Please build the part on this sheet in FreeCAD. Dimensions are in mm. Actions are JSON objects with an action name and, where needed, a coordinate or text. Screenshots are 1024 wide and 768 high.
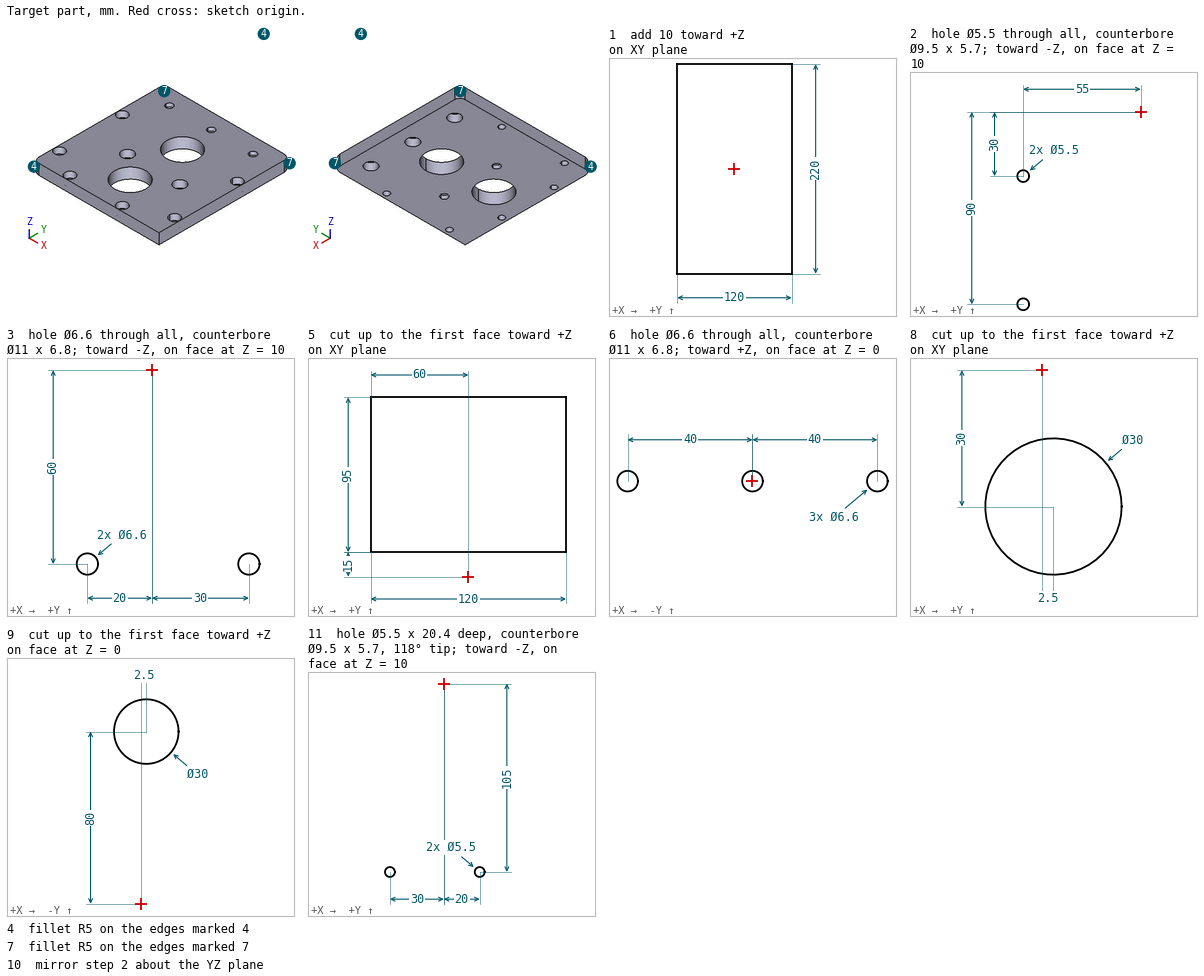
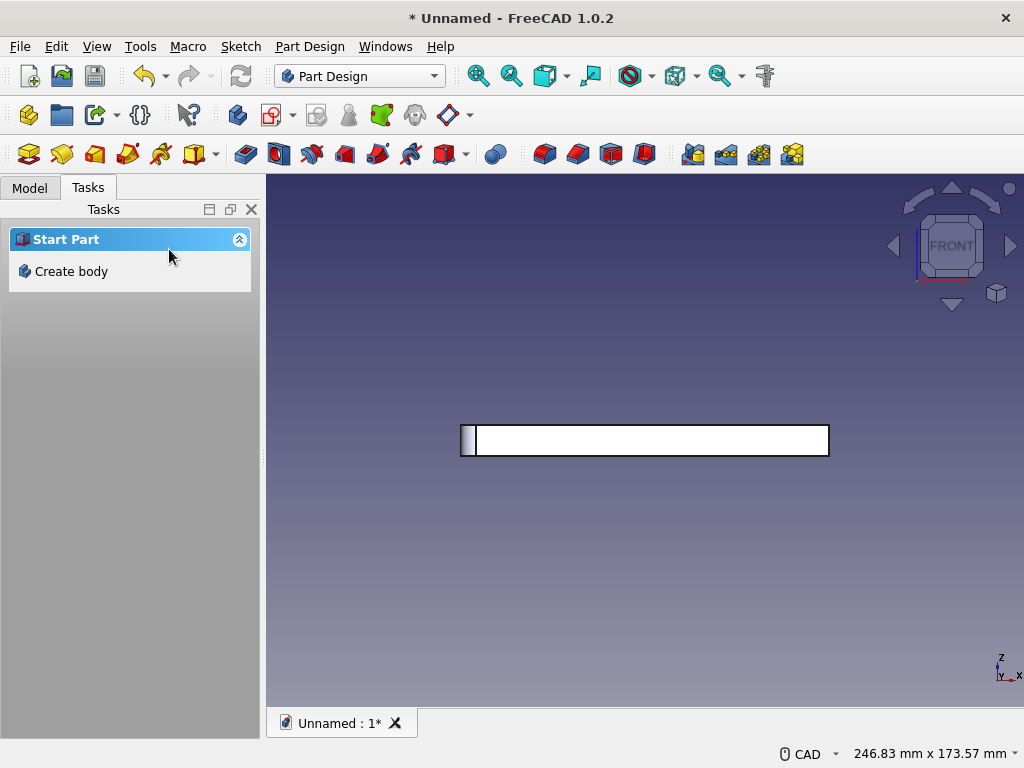
{"action": "key", "text": "3"}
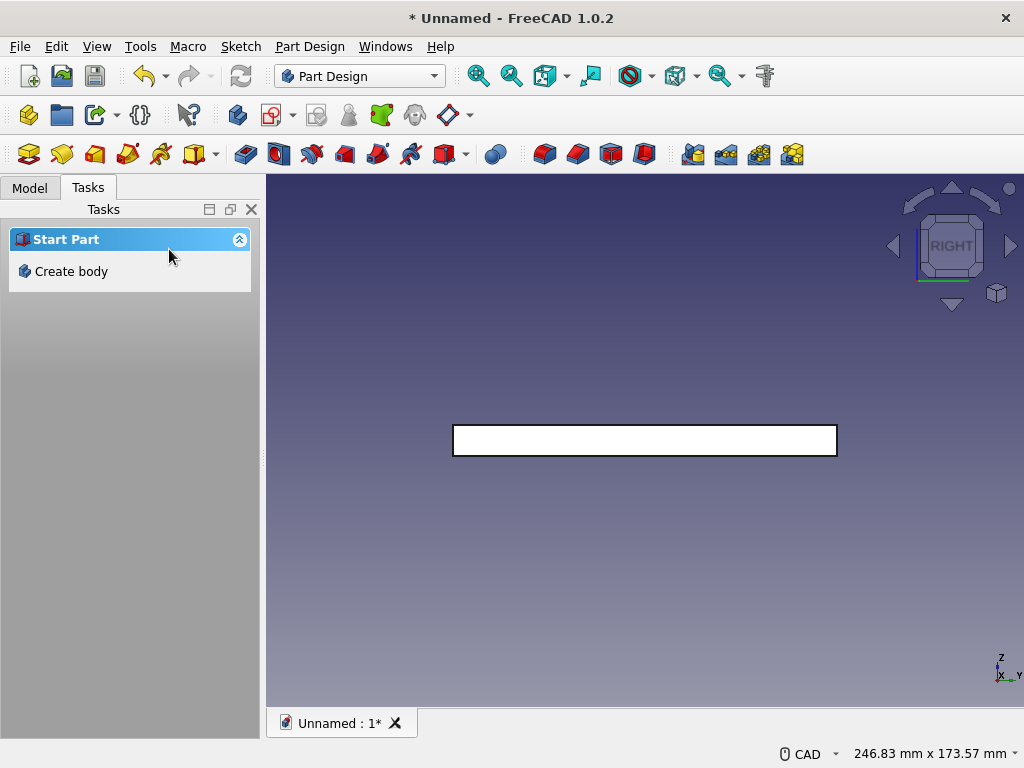
{"action": "left_click", "coordinate": [837, 439]}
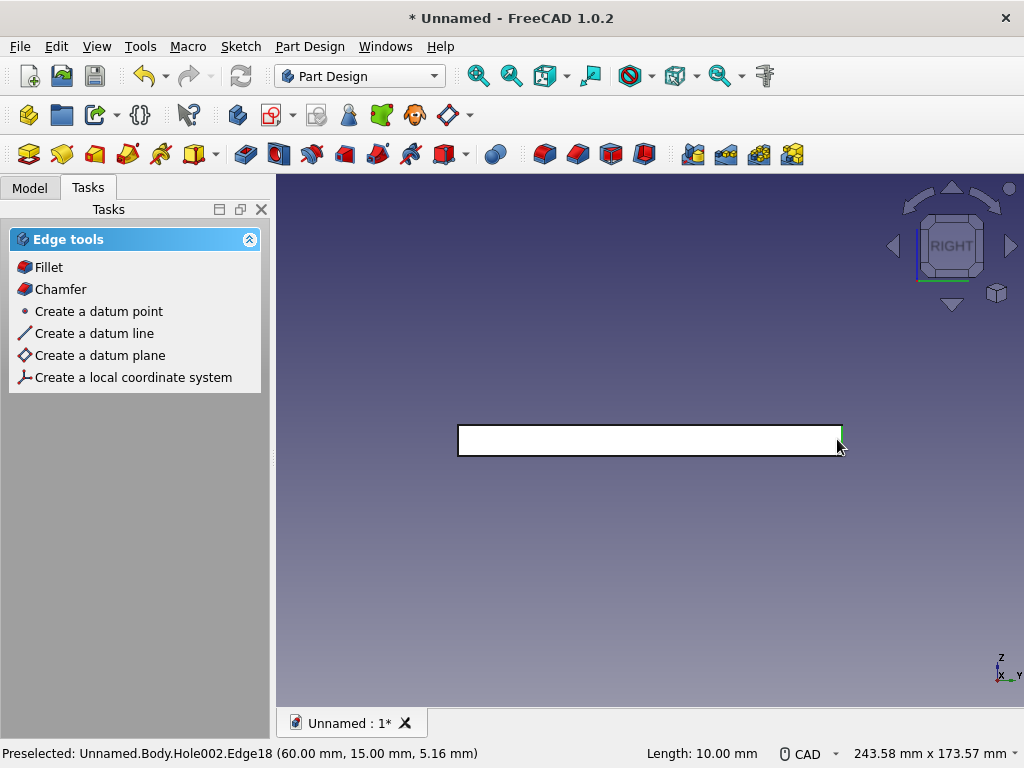
{"action": "key", "text": "5"}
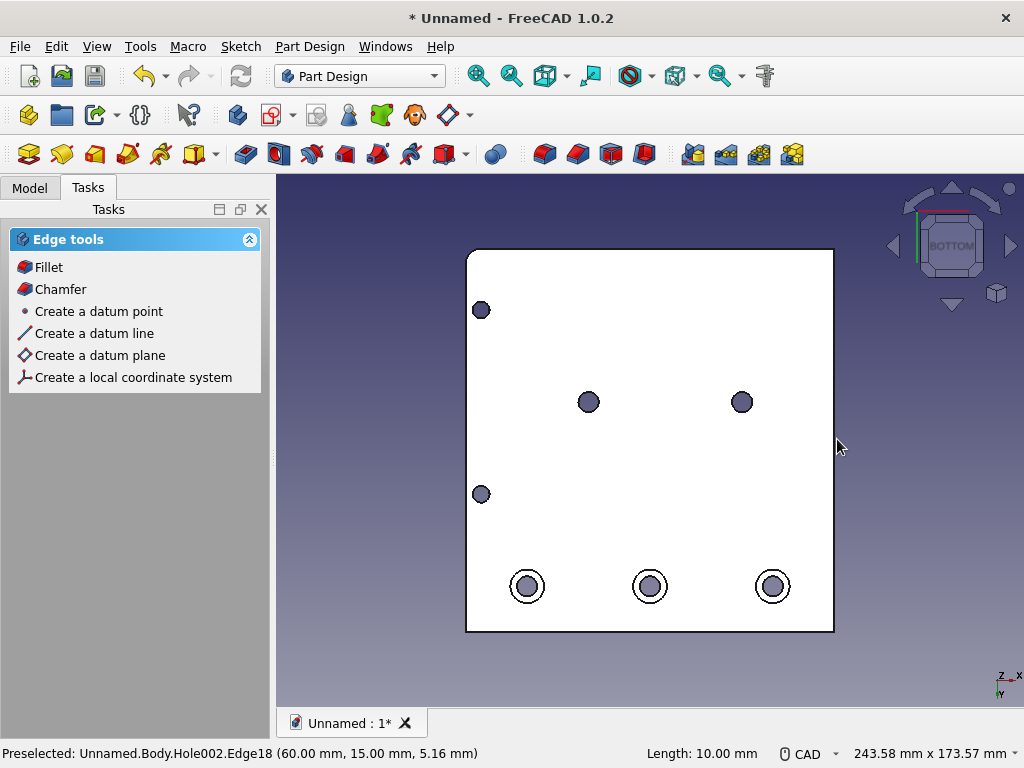
{"action": "key", "text": "4"}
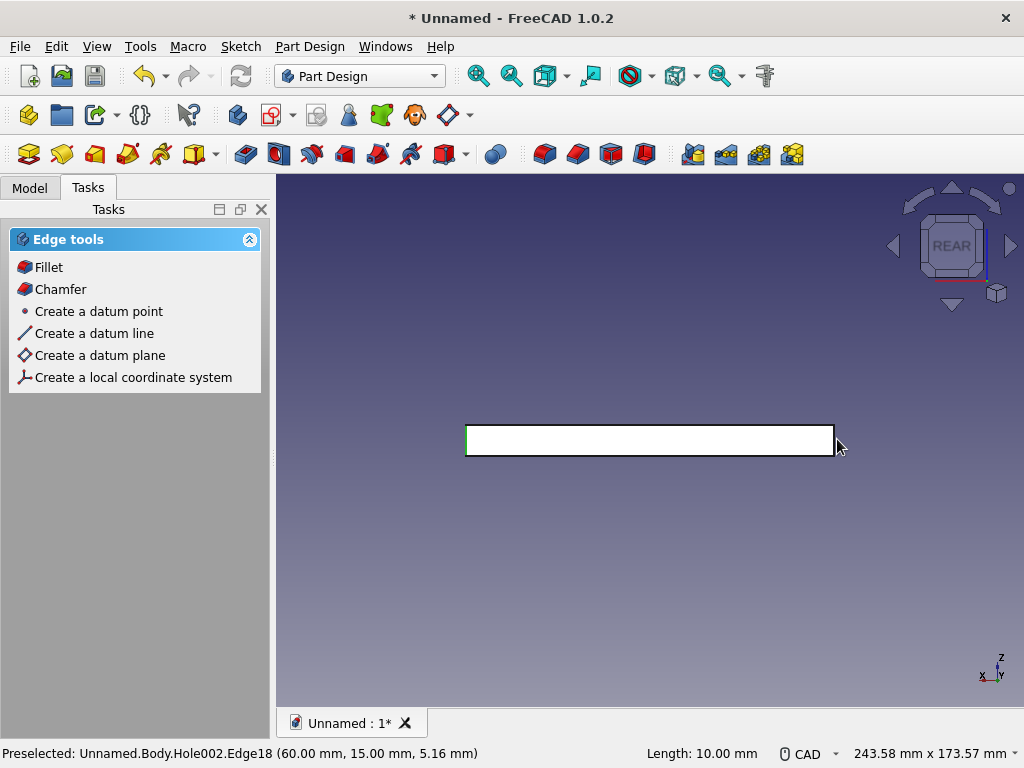
{"action": "left_click", "coordinate": [834, 439], "text": "ctrl"}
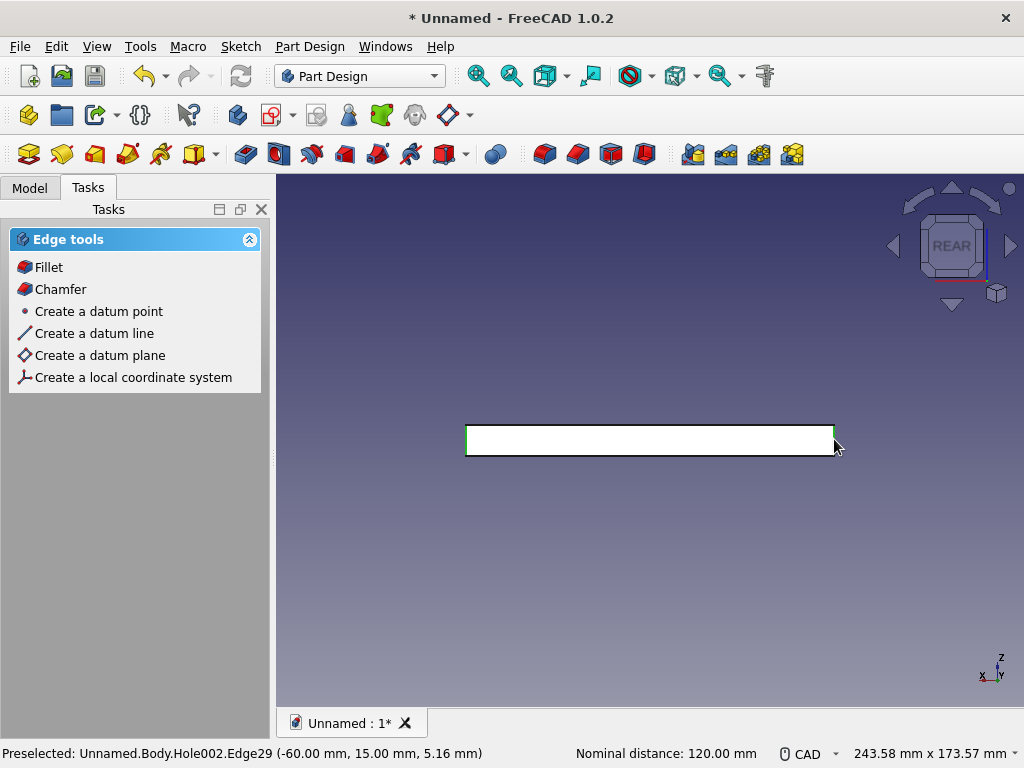
{"action": "left_click", "coordinate": [545, 154]}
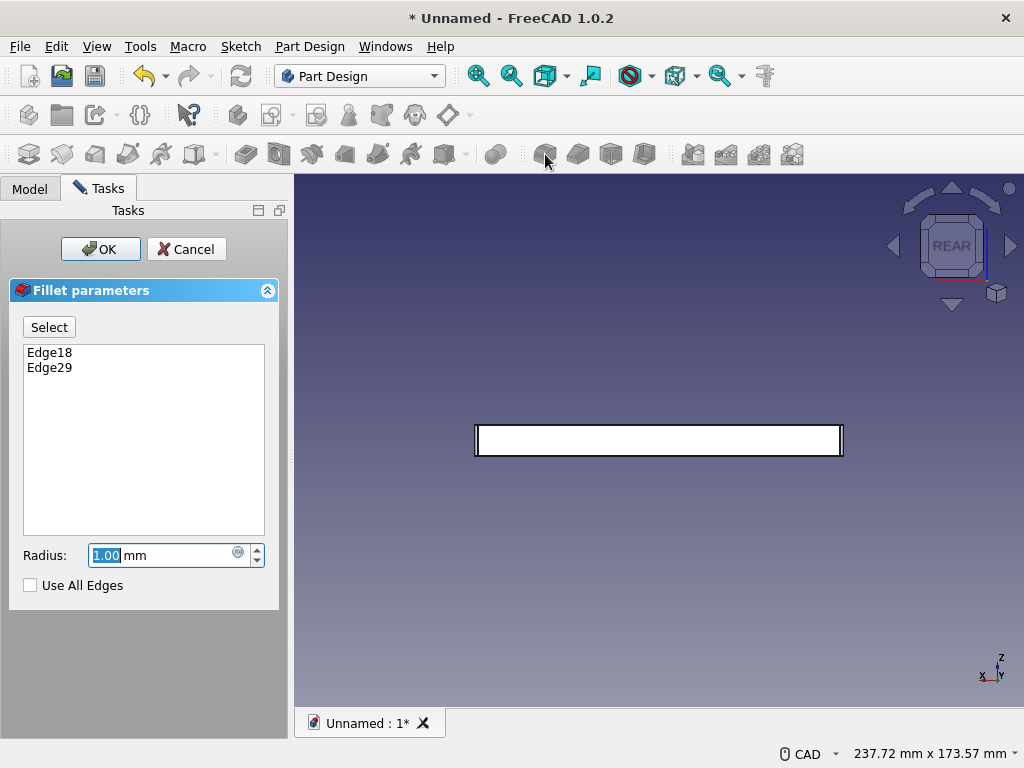
{"action": "type", "text": "5"}
{"action": "key", "text": "Tab"}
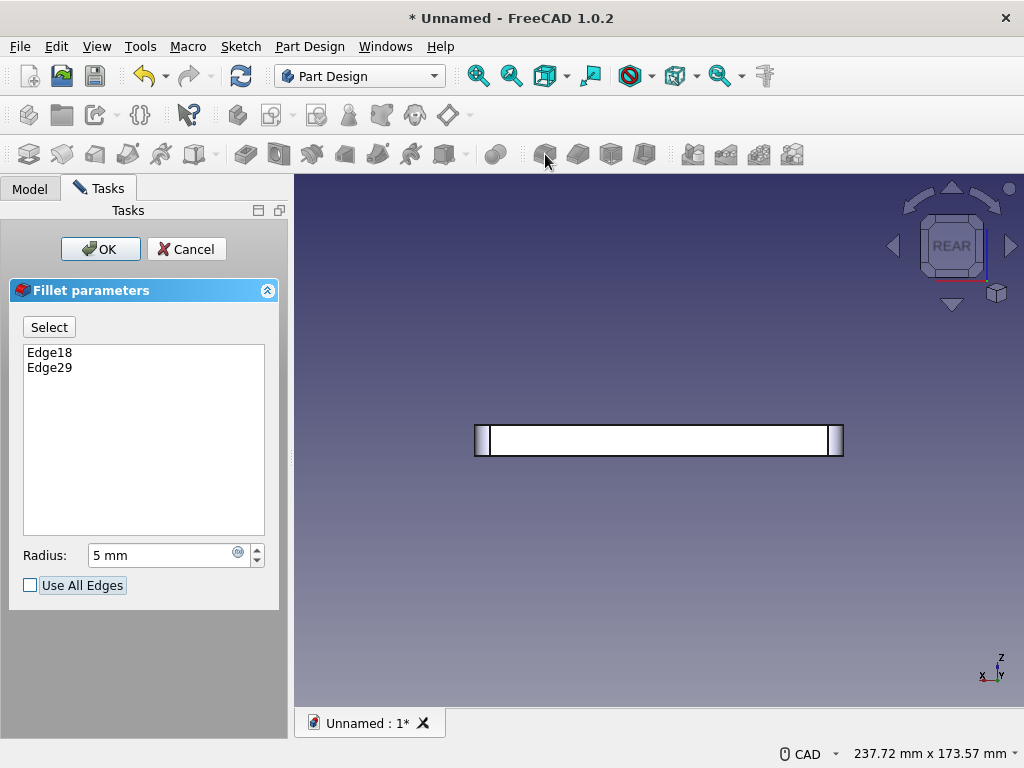
{"action": "left_click", "coordinate": [101, 249]}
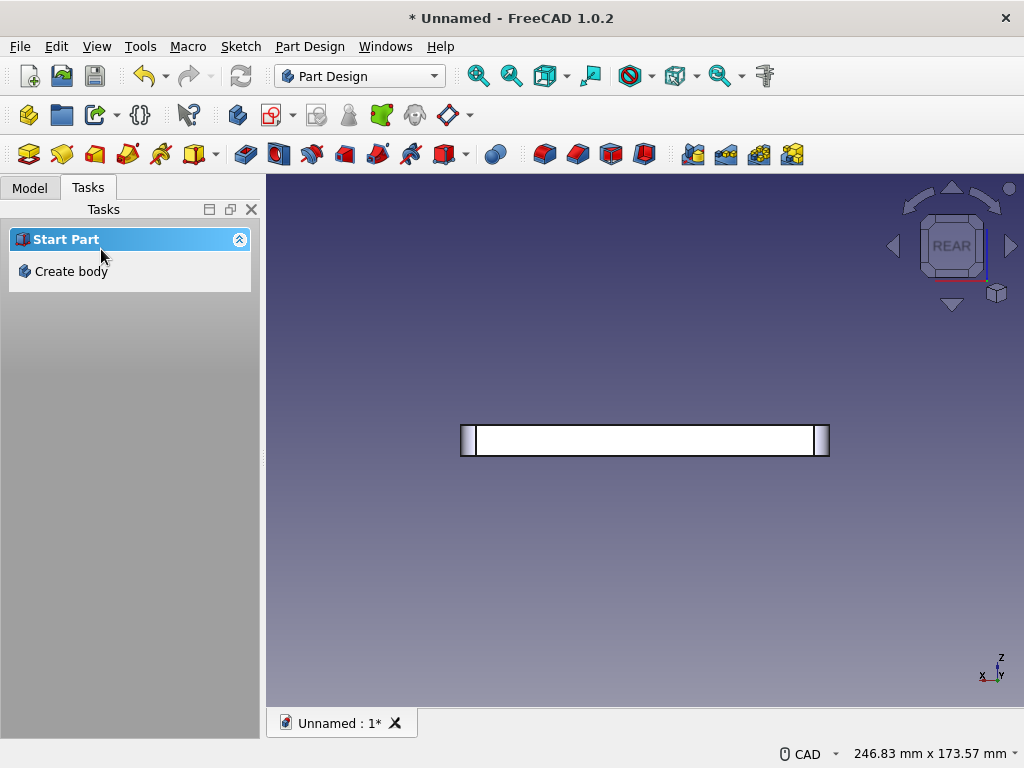
{"action": "left_click", "coordinate": [270, 116]}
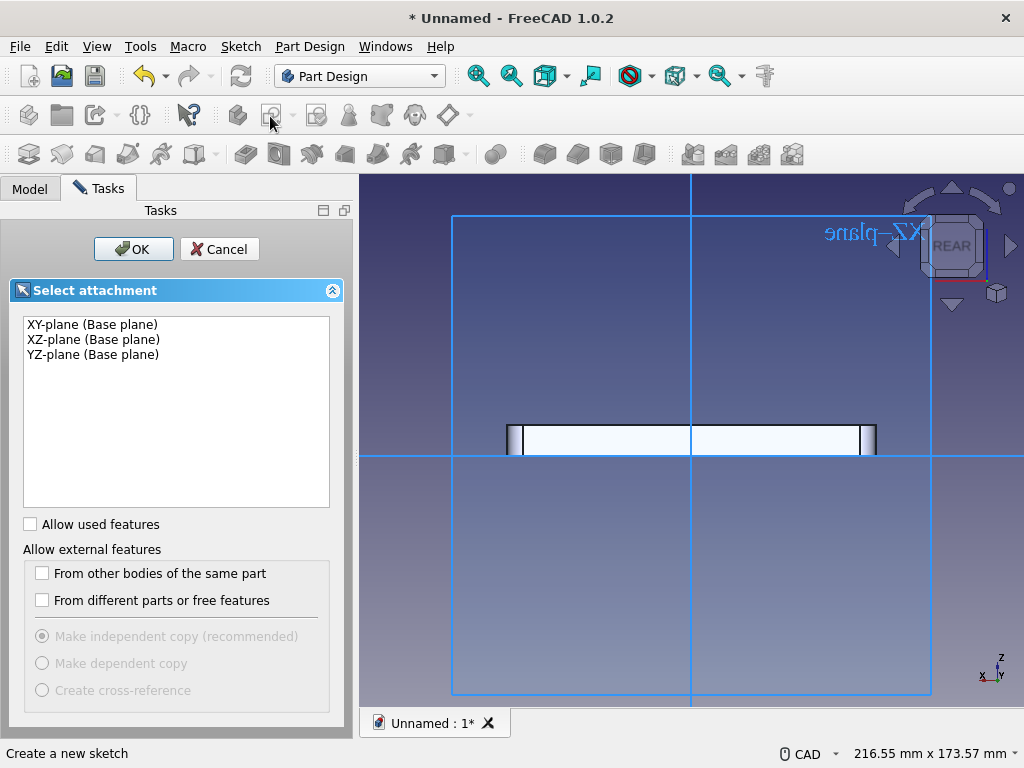
{"action": "left_click", "coordinate": [84, 324]}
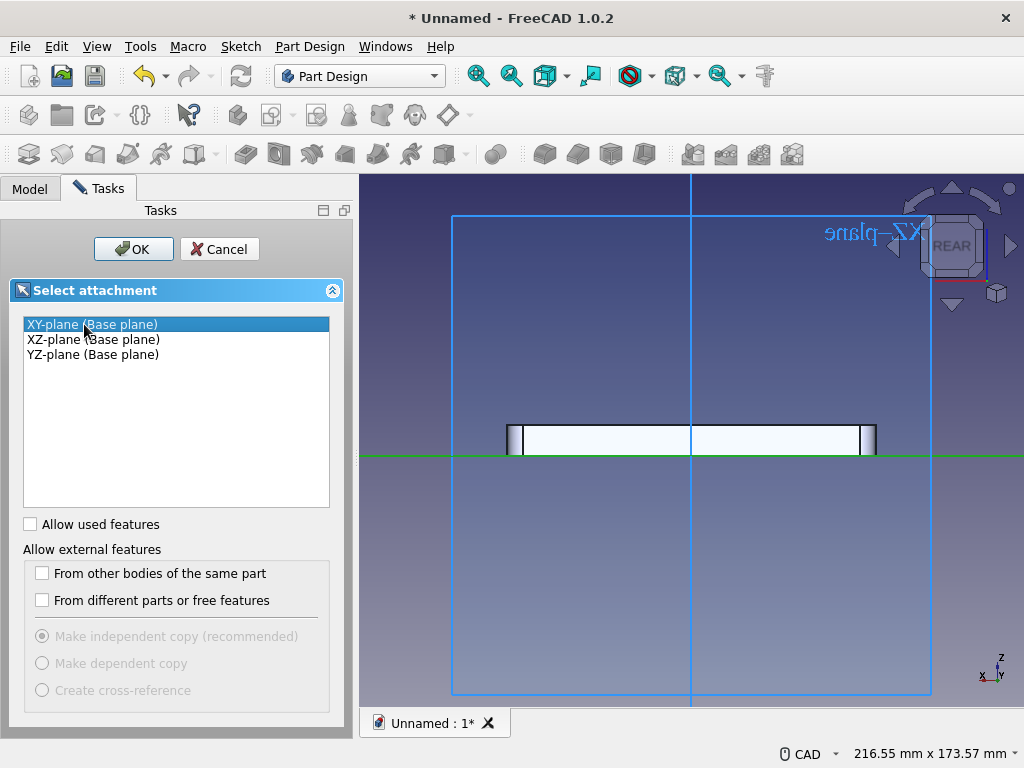
{"action": "left_click", "coordinate": [134, 249]}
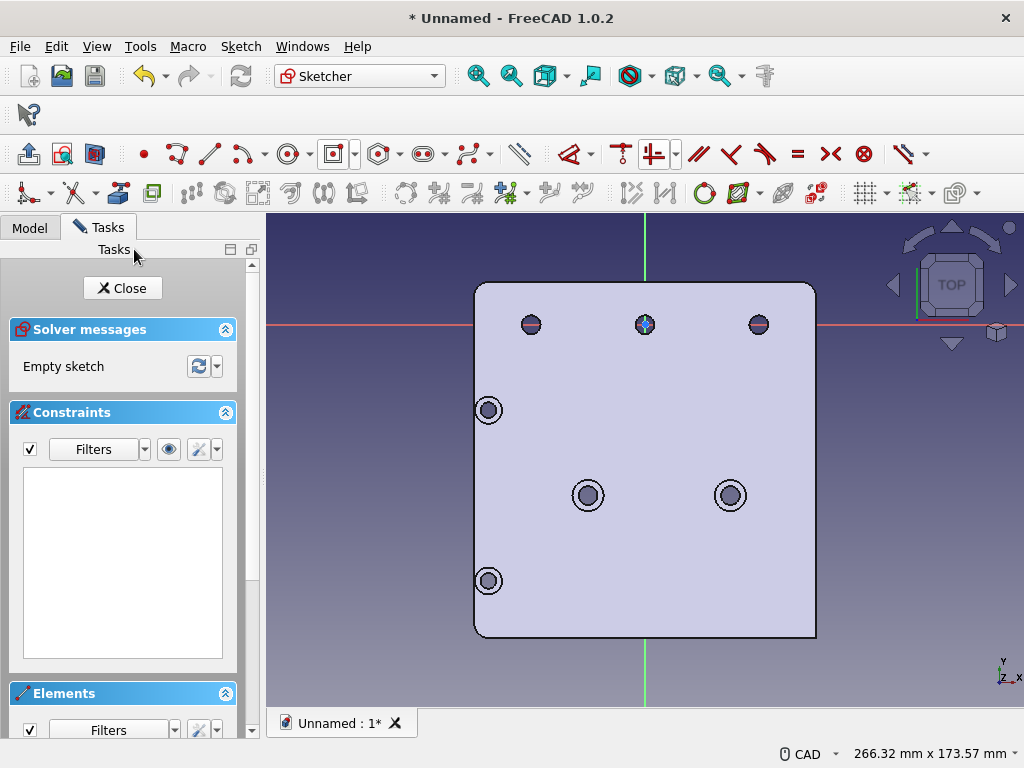
{"action": "left_click", "coordinate": [95, 154]}